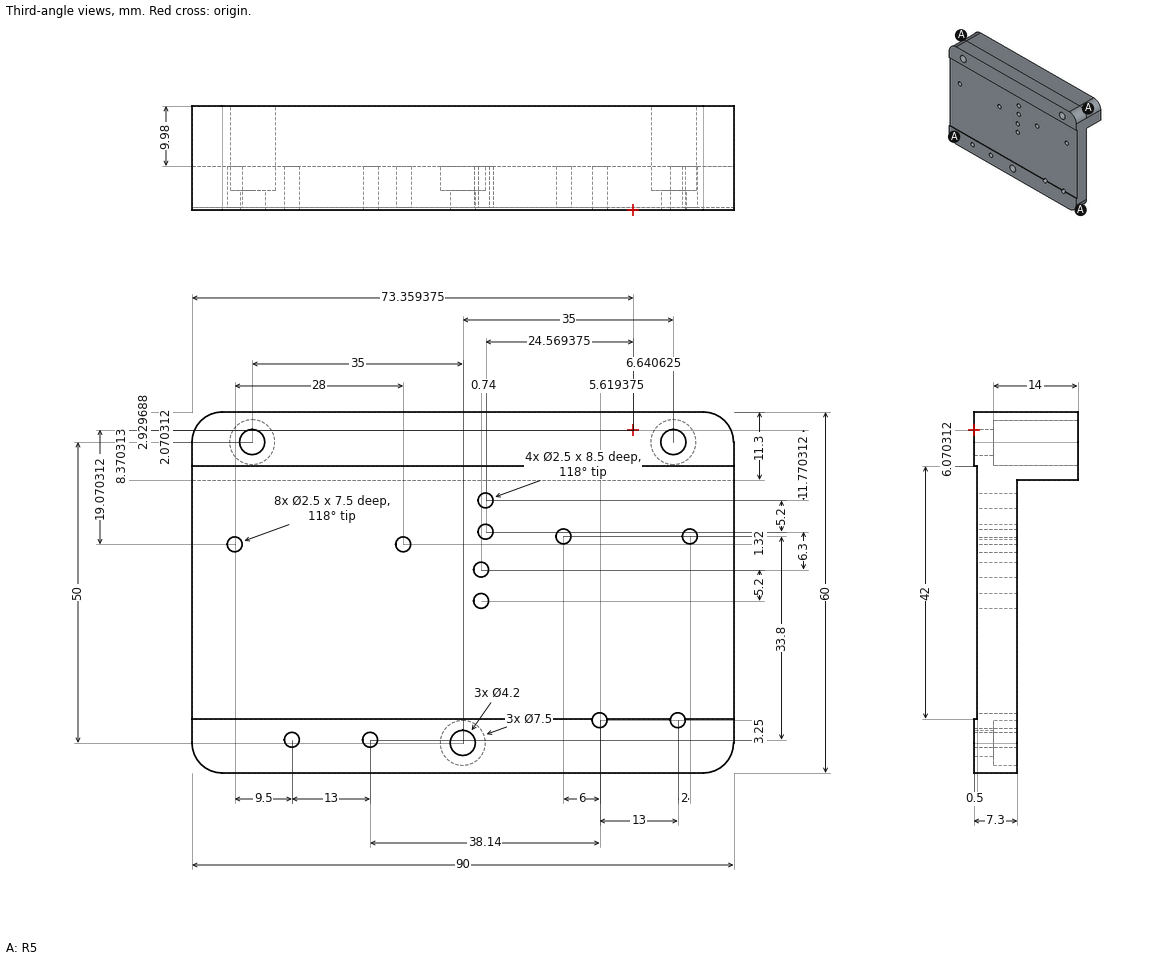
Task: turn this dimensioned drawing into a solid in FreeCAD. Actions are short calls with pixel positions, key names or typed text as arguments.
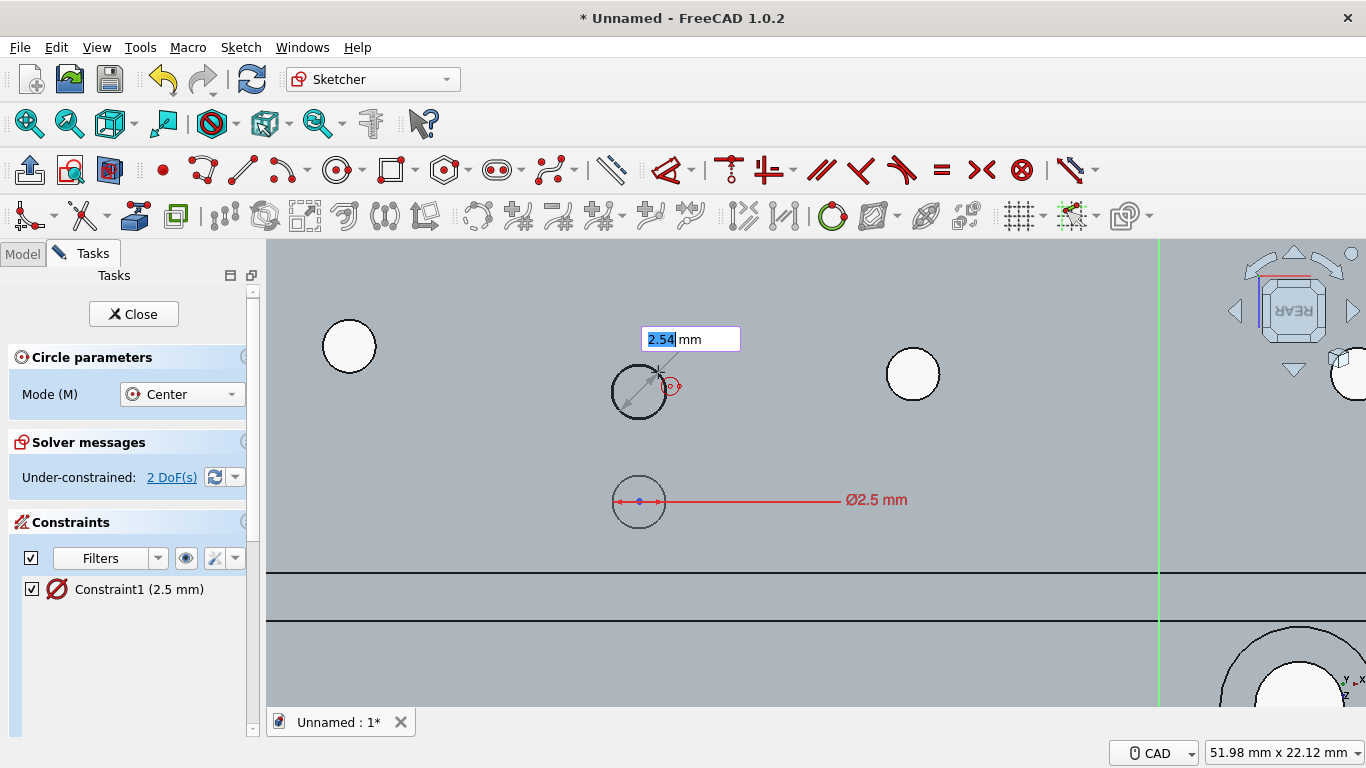
text(2.5)
key(Return)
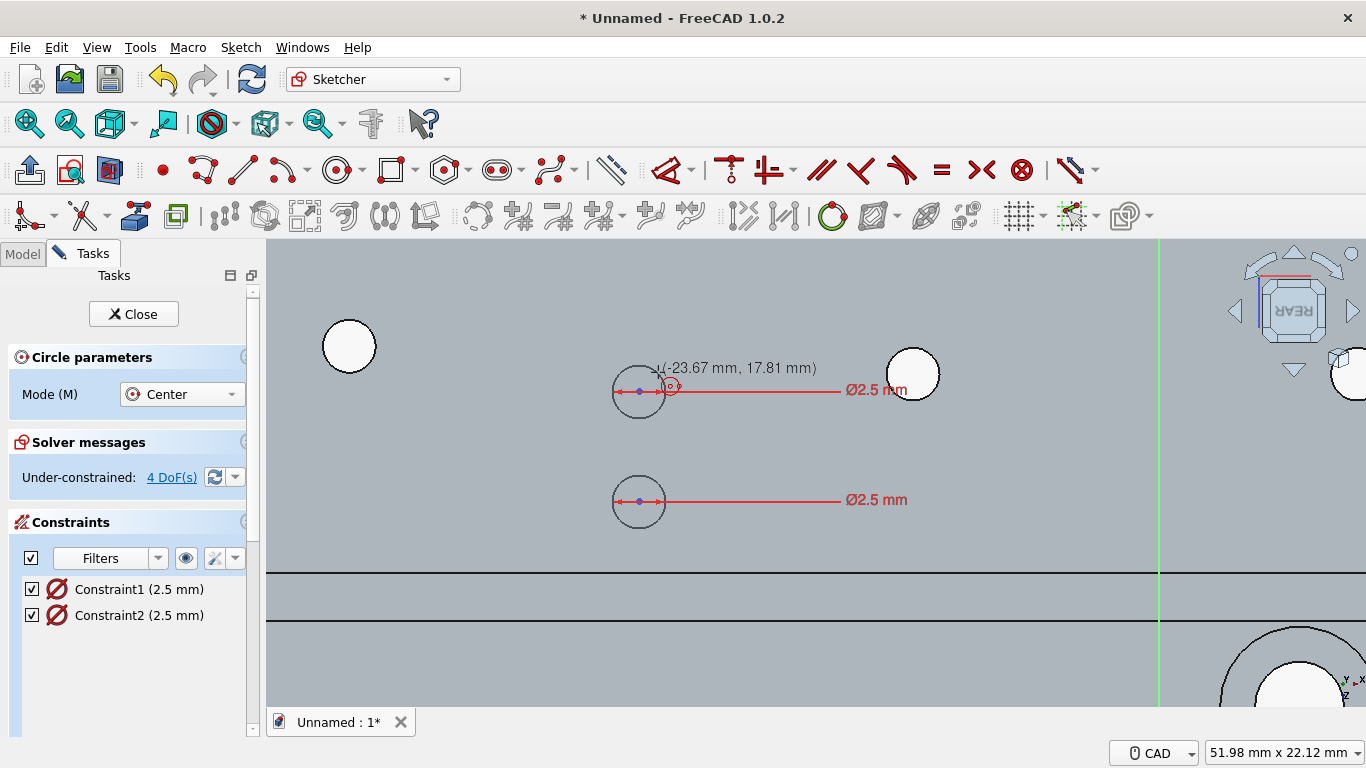
scroll(641, 504, down, 4)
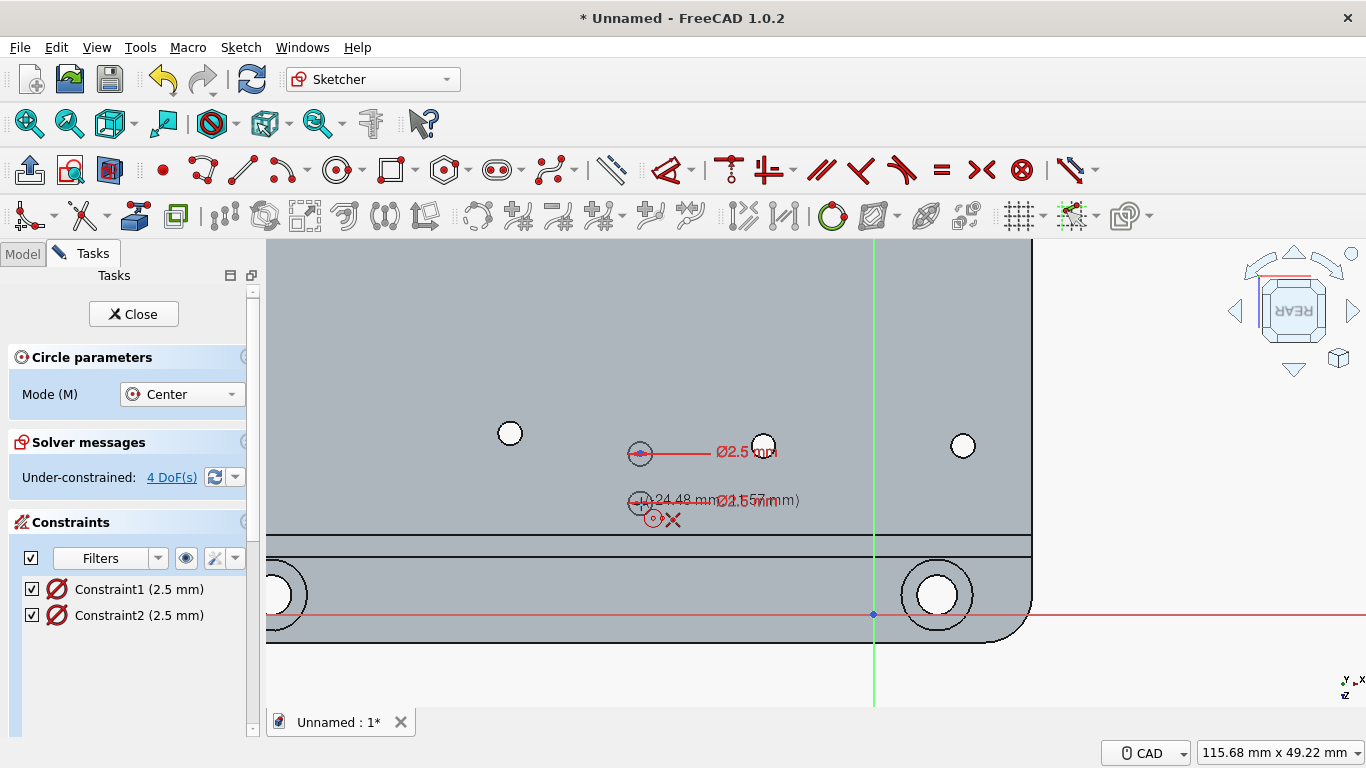
scroll(633, 393, up, 4)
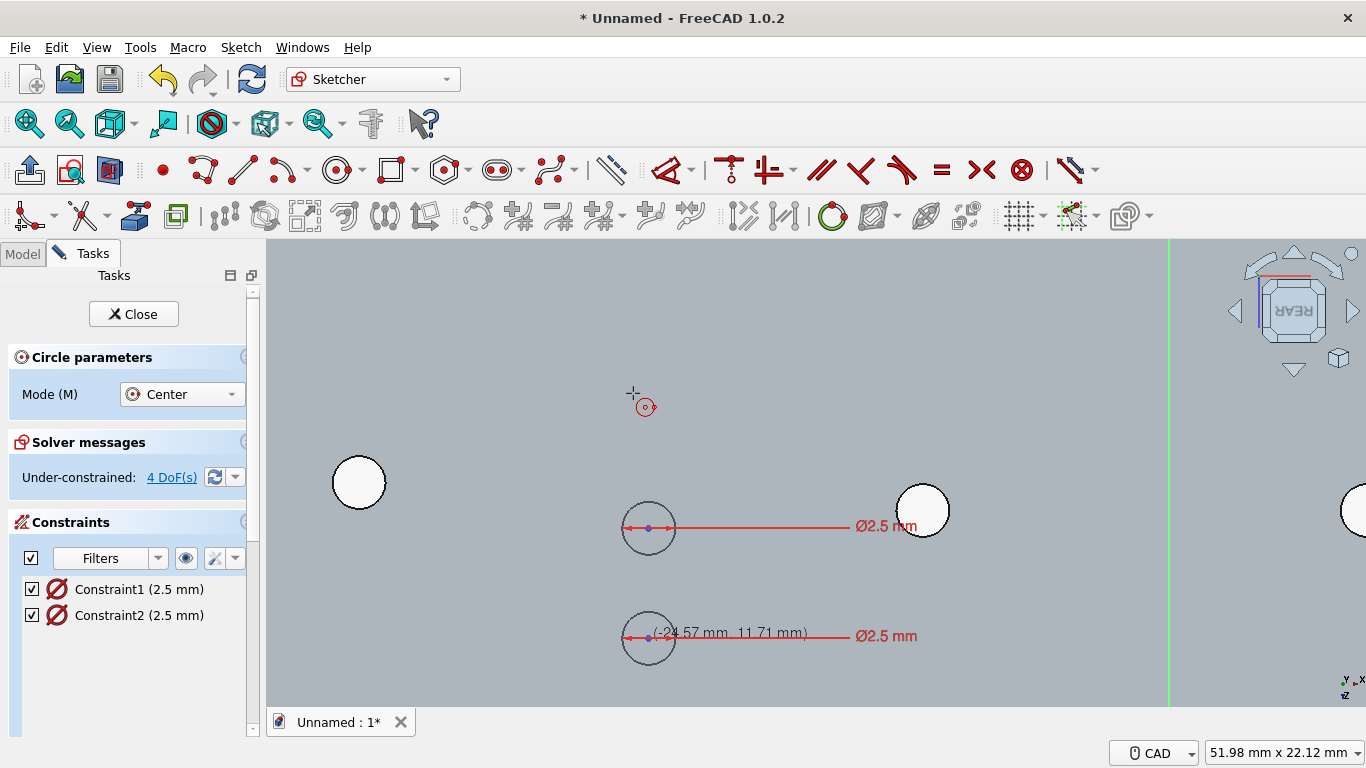
click(633, 394)
move(652, 375)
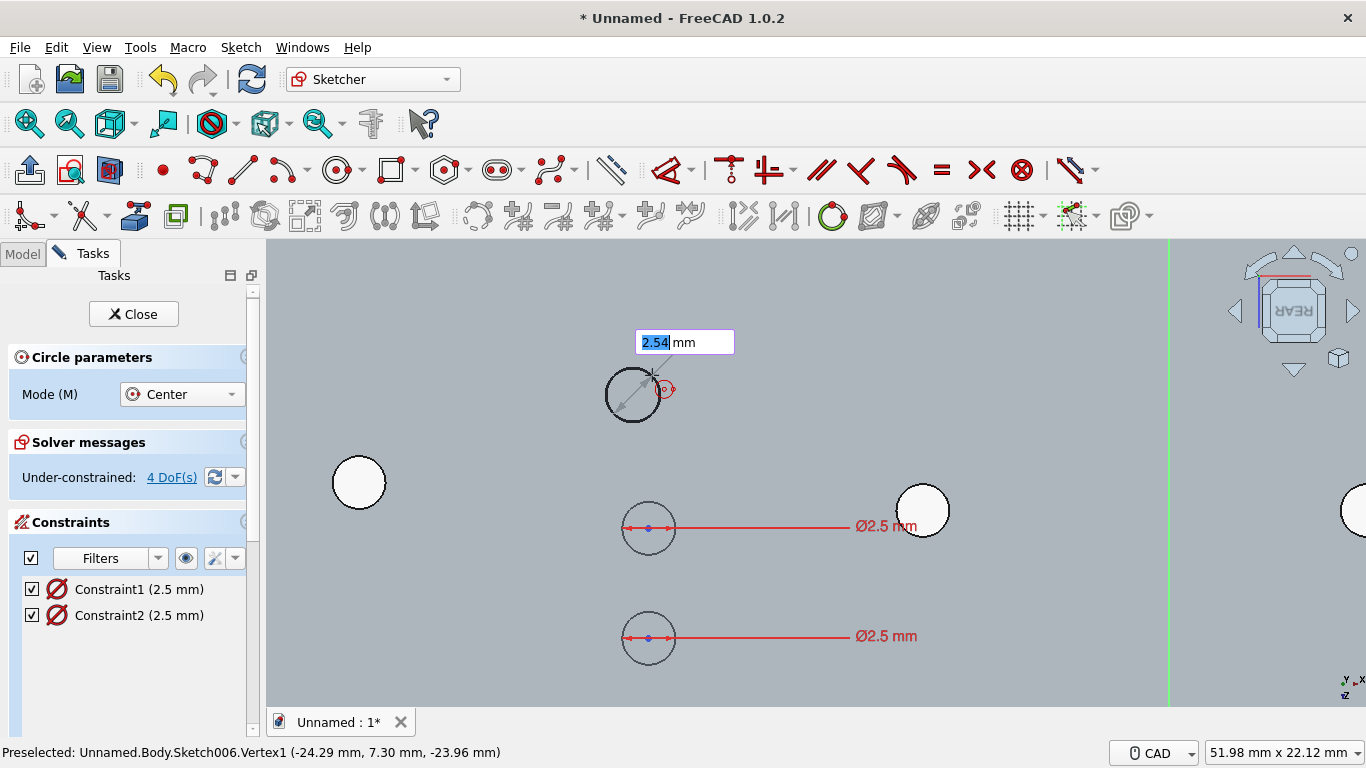
text(2.5)
key(Return)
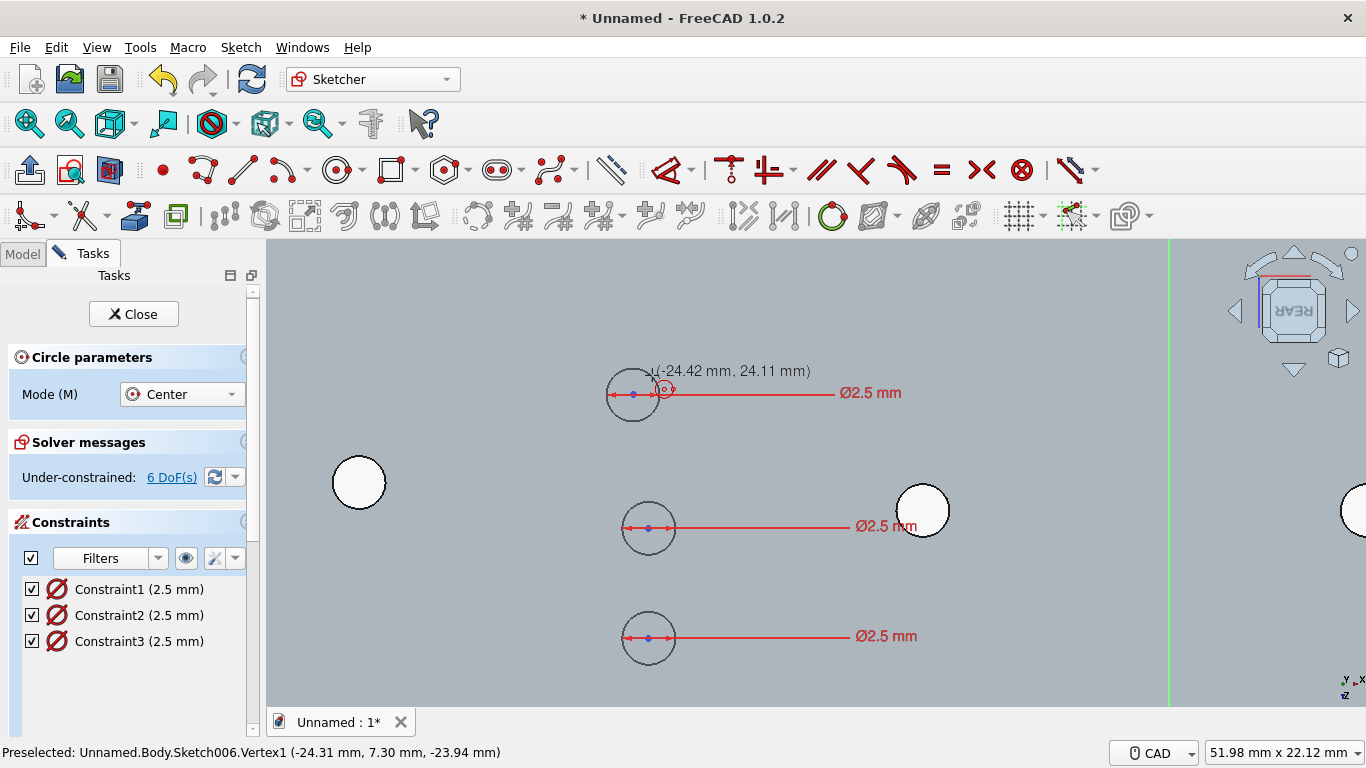
click(633, 284)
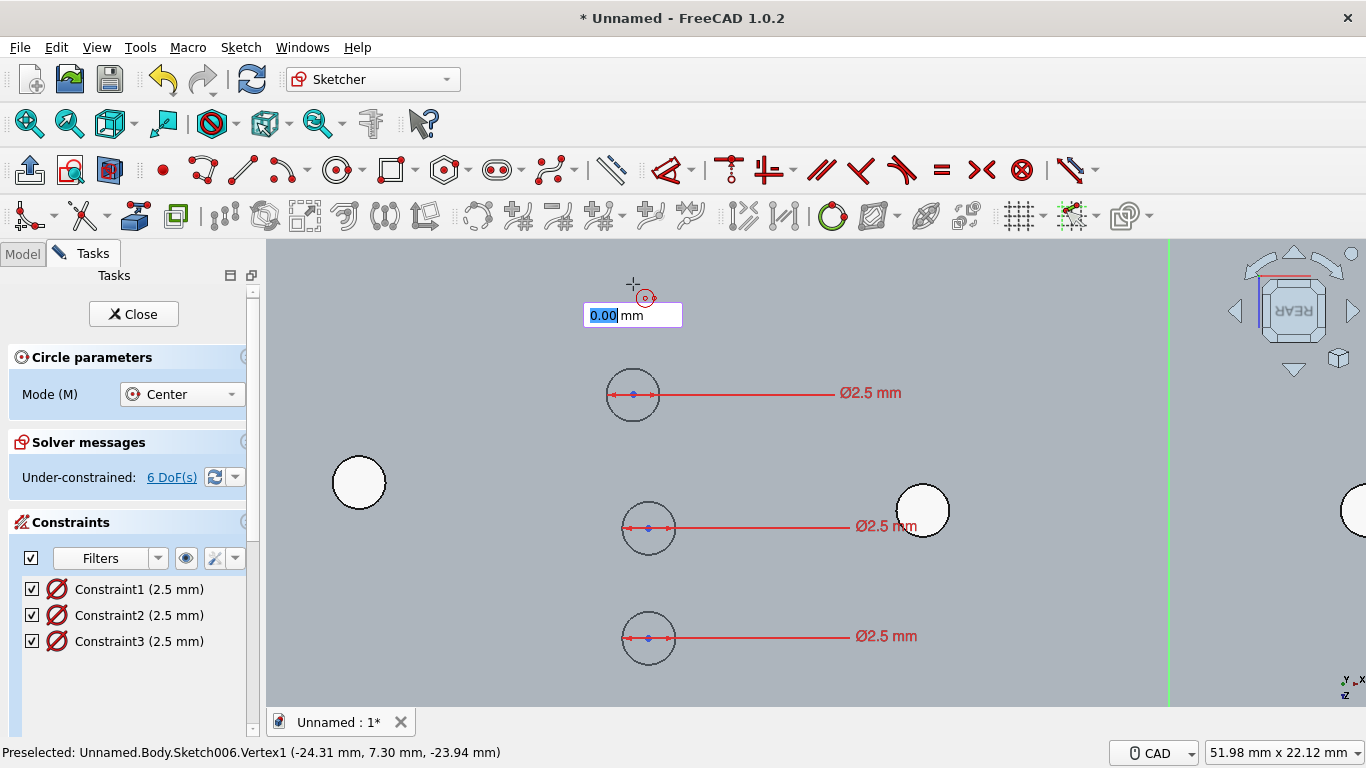
scroll(633, 392, down, 4)
move(642, 335)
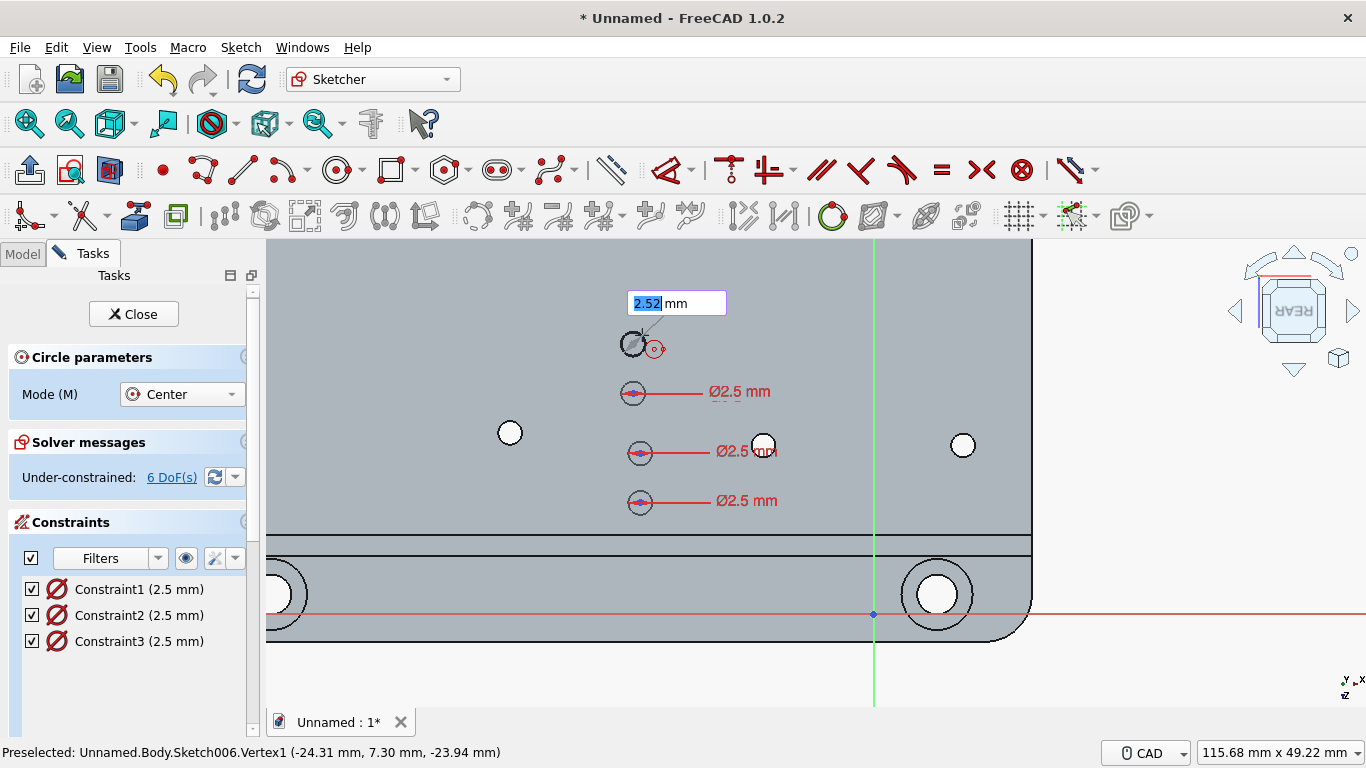
text(2.5)
key(Return)
key(Escape)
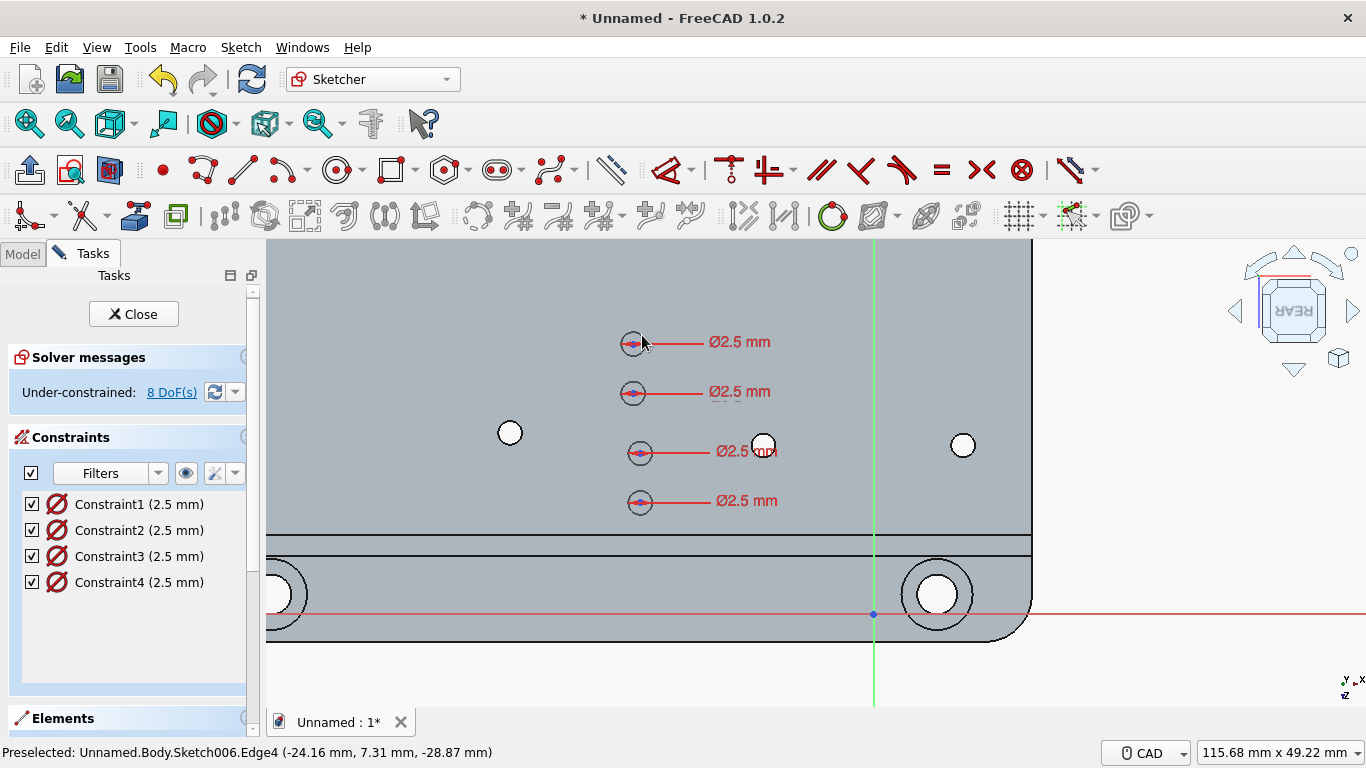
click(666, 170)